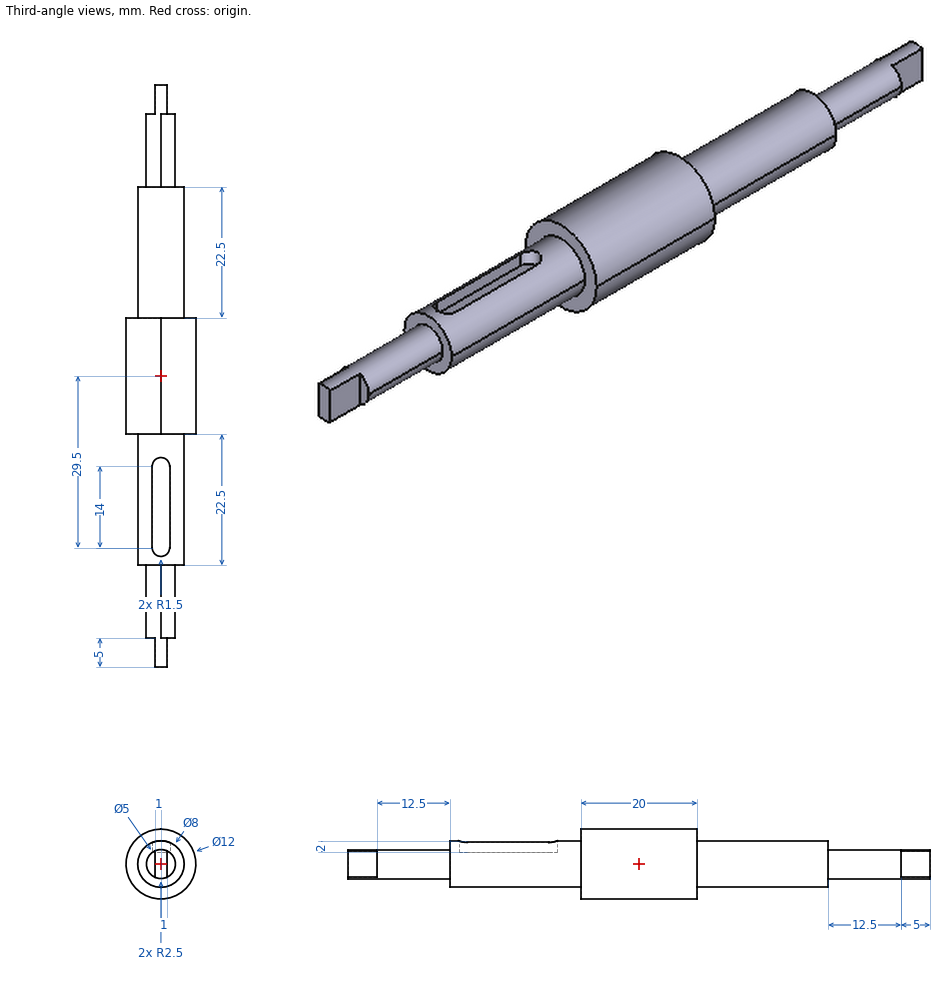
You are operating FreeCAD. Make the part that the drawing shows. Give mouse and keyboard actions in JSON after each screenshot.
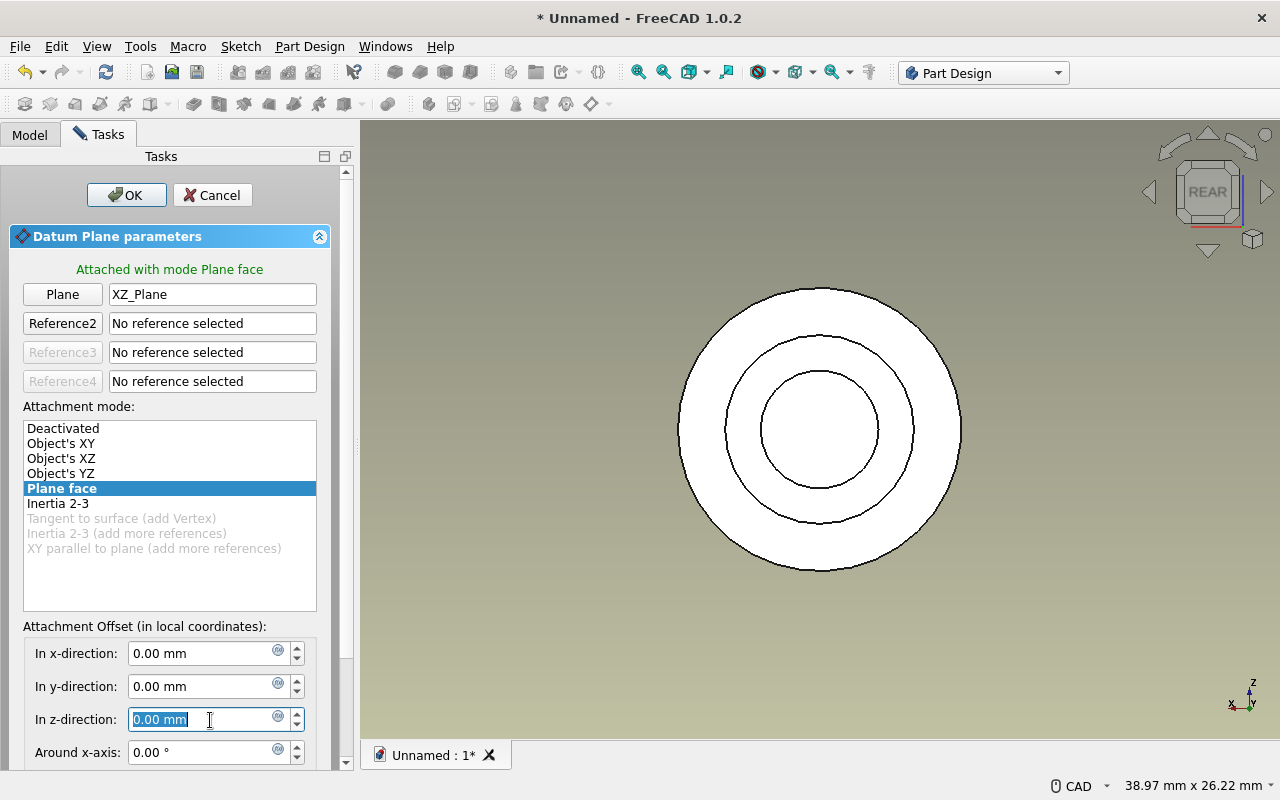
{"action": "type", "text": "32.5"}
{"action": "key", "text": "Tab"}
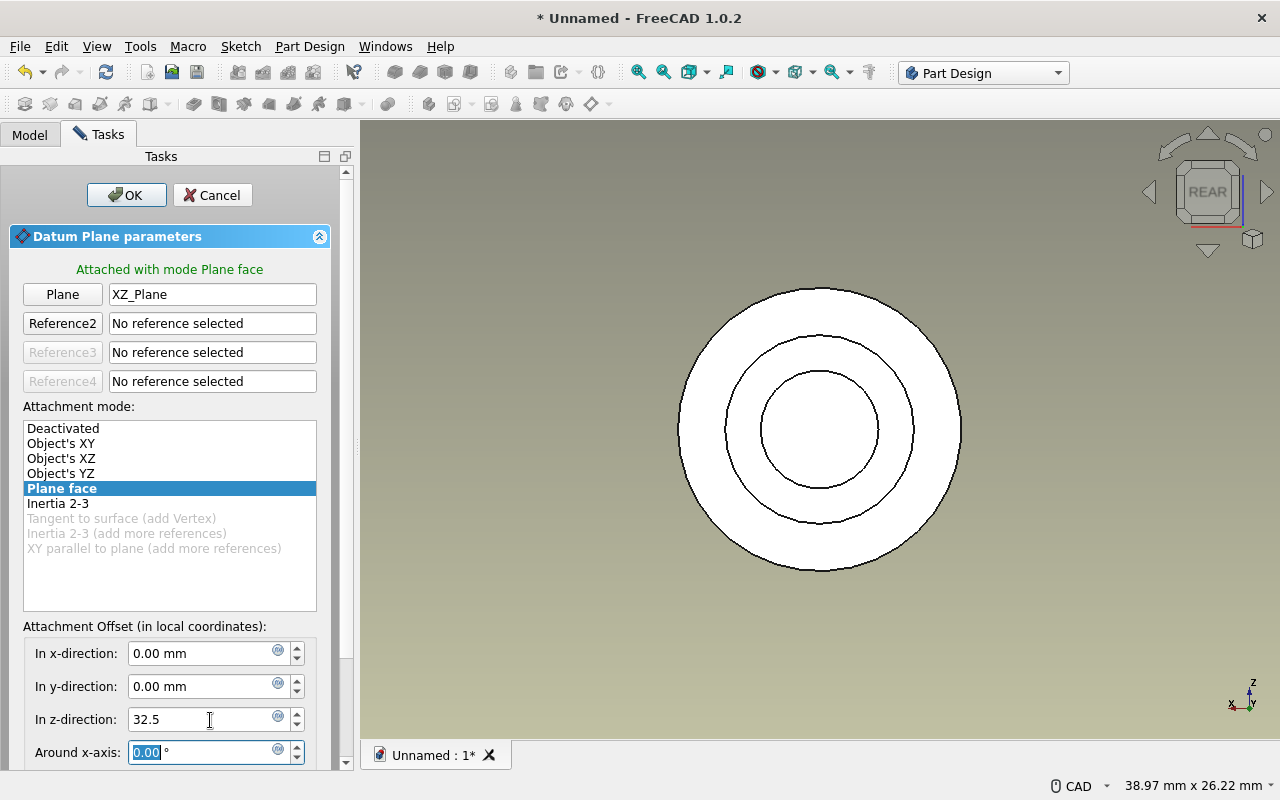
{"action": "left_click", "coordinate": [127, 195]}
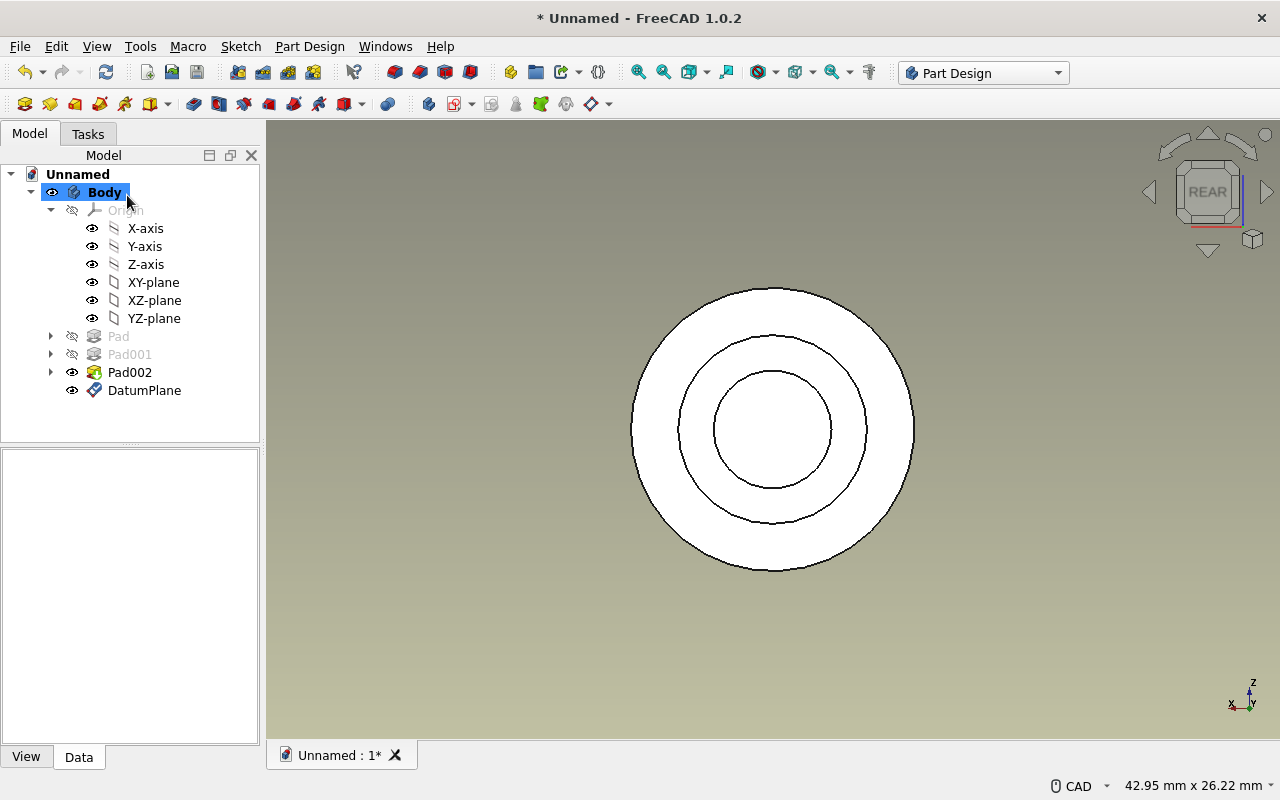
{"action": "left_click", "coordinate": [117, 390]}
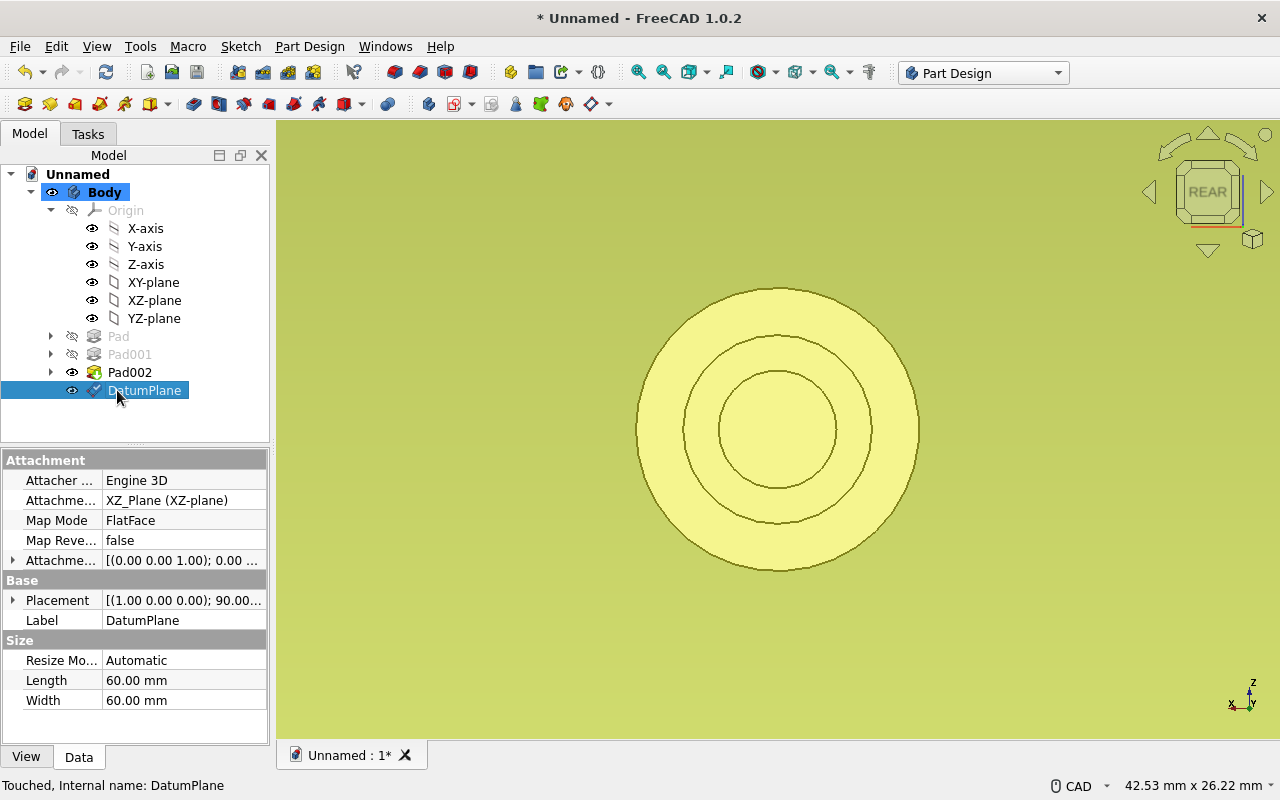
{"action": "left_click", "coordinate": [454, 104]}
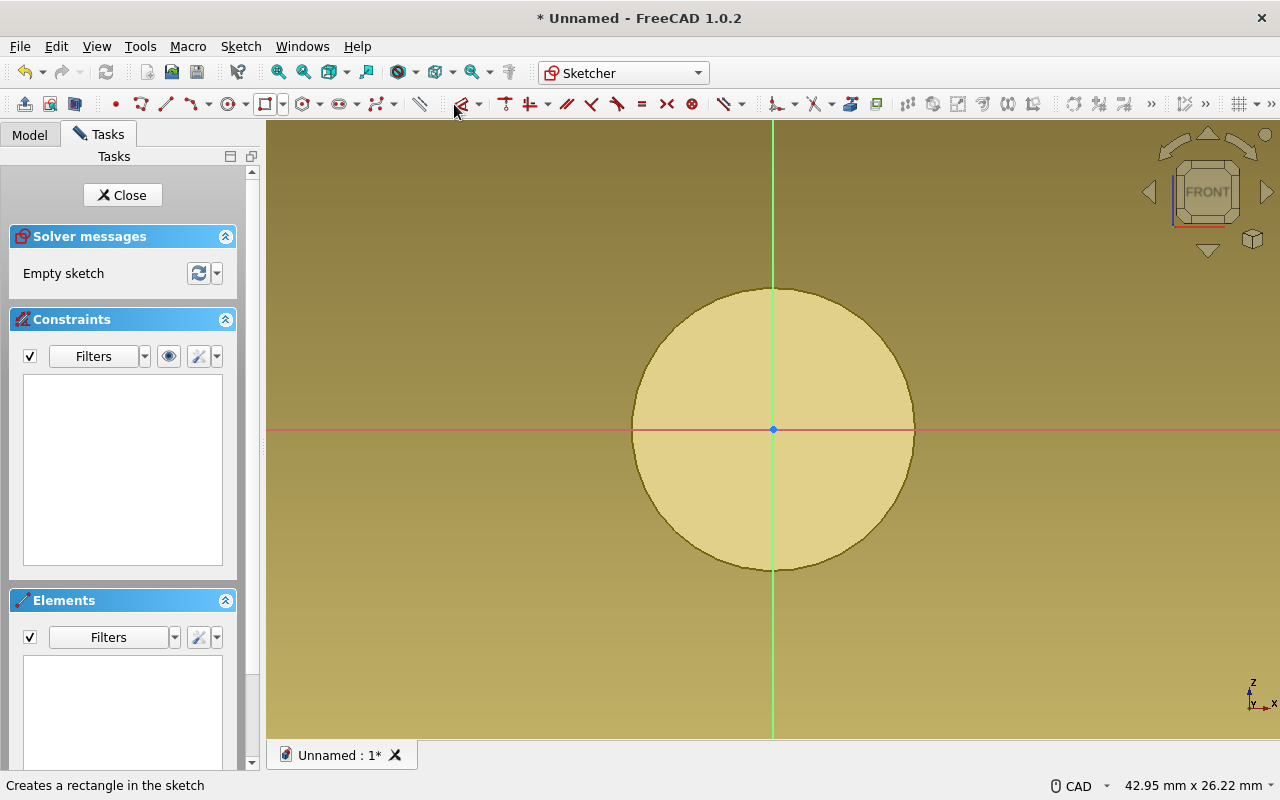
{"action": "scroll", "coordinate": [830, 429], "scroll_direction": "up", "scroll_amount": 4}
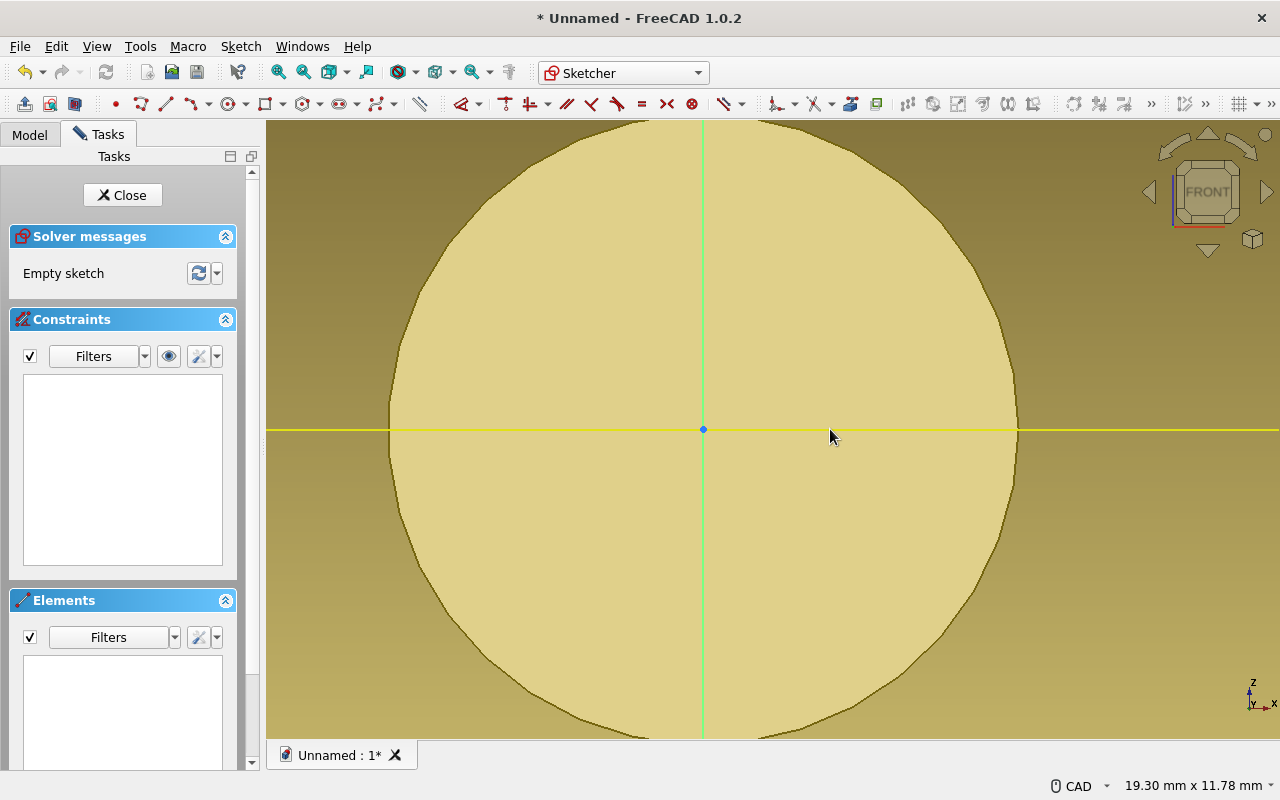
{"action": "left_click", "coordinate": [228, 104]}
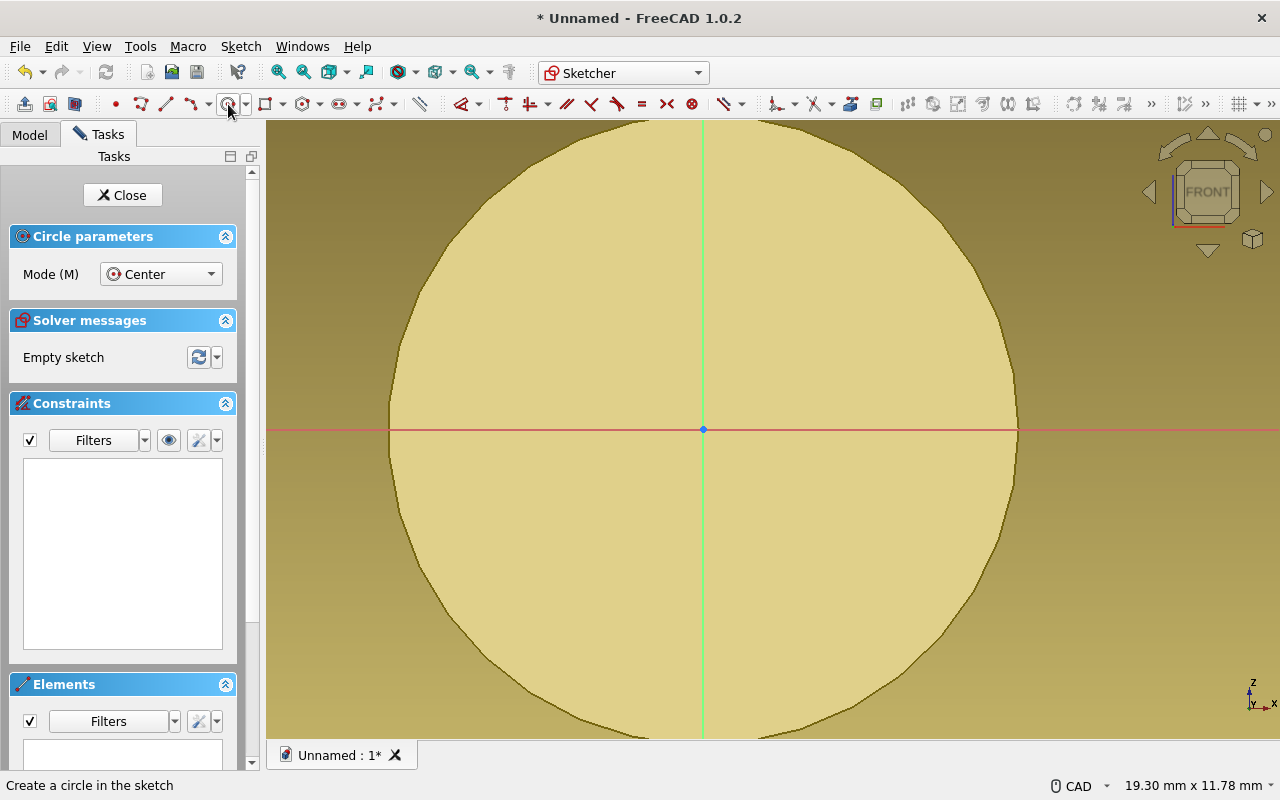
{"action": "left_click", "coordinate": [703, 429]}
{"action": "mouse_move", "coordinate": [852, 281]}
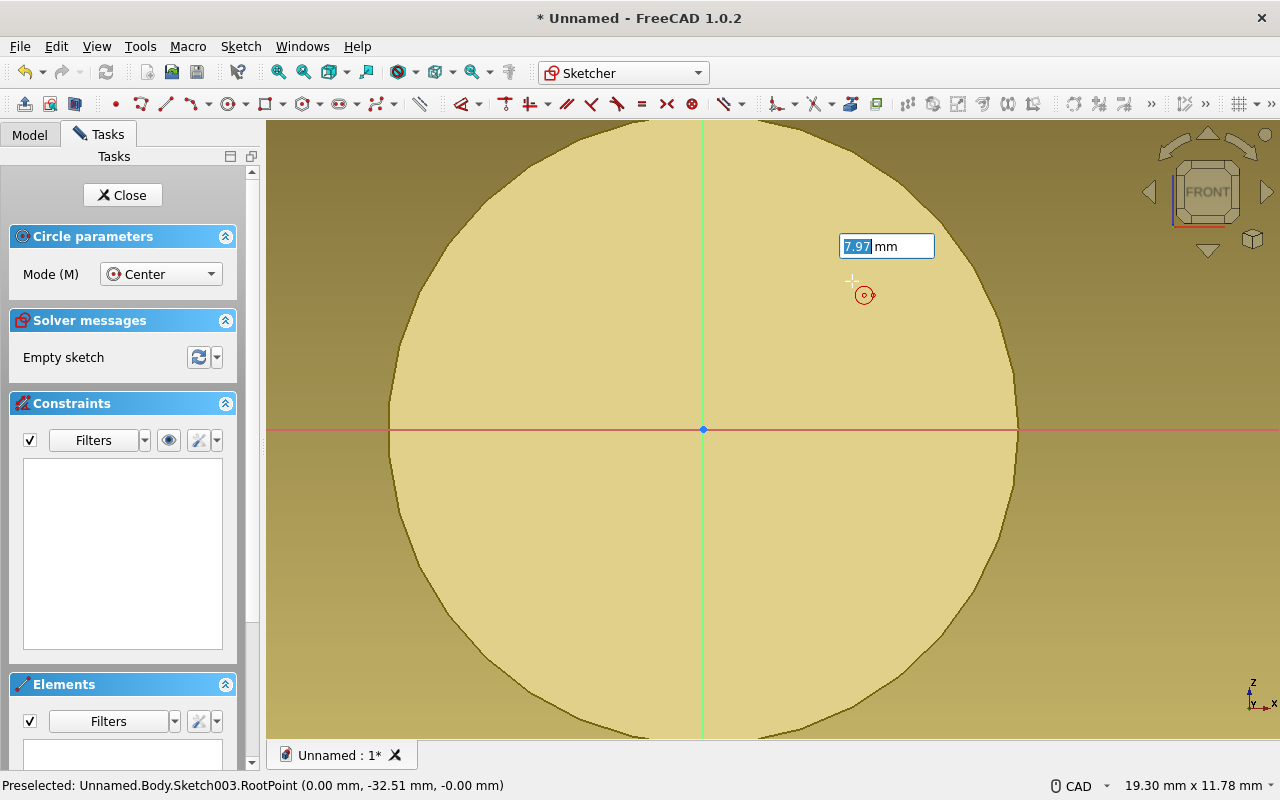
{"action": "type", "text": "8"}
{"action": "key", "text": "Return"}
{"action": "key", "text": "Escape"}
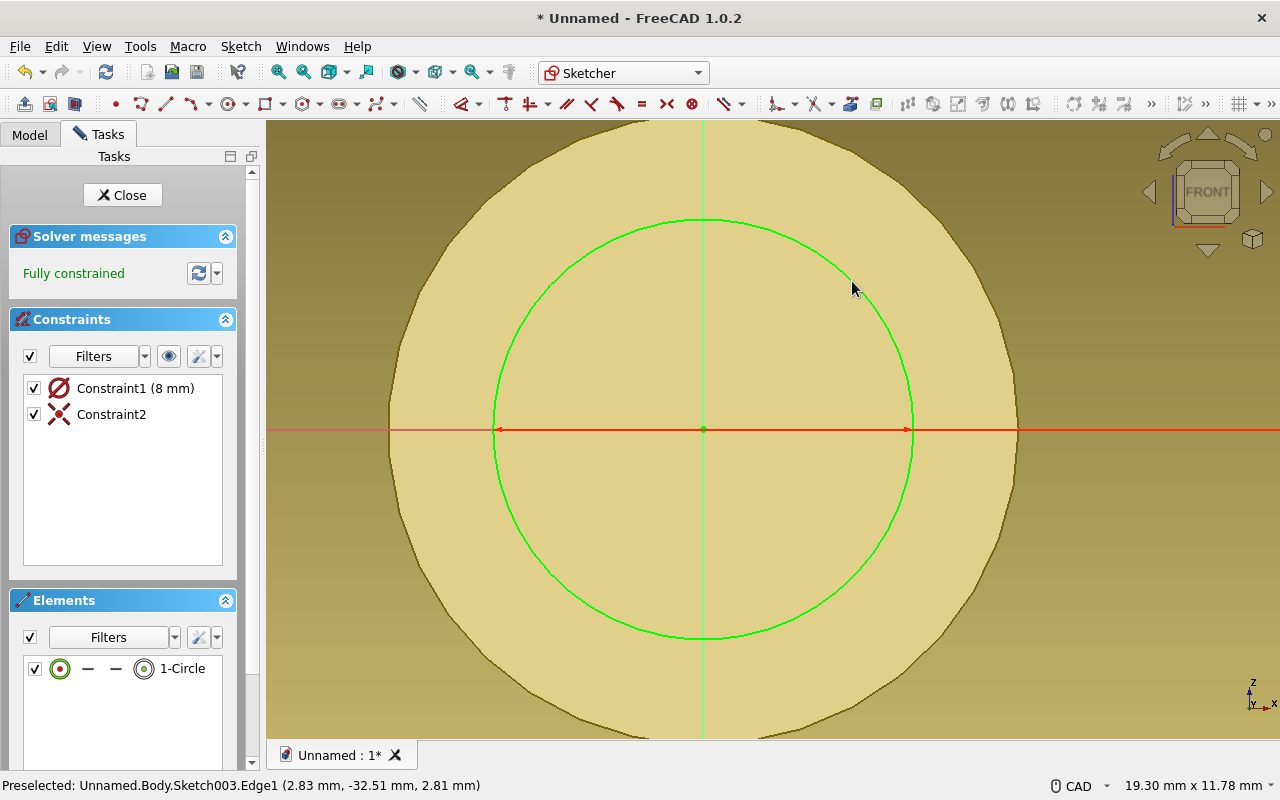
{"action": "left_click", "coordinate": [123, 195]}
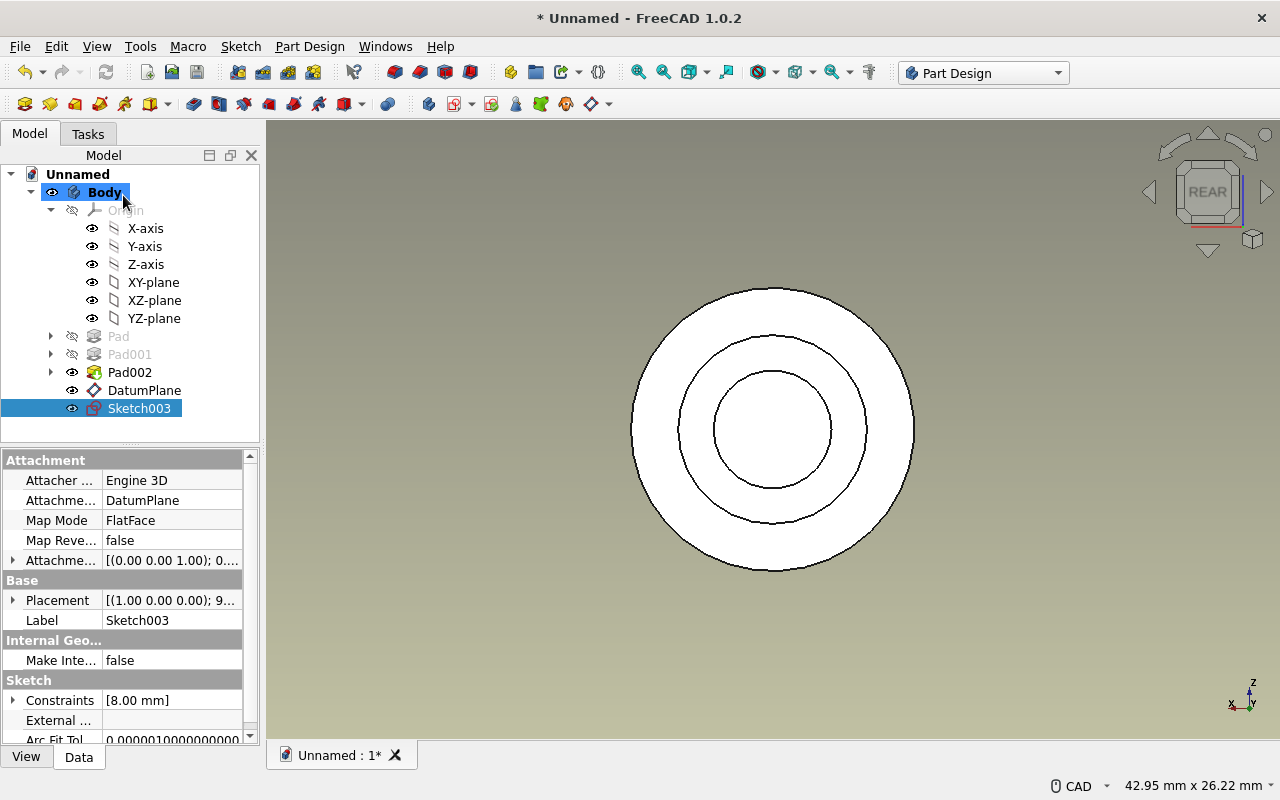
{"action": "left_click", "coordinate": [25, 104]}